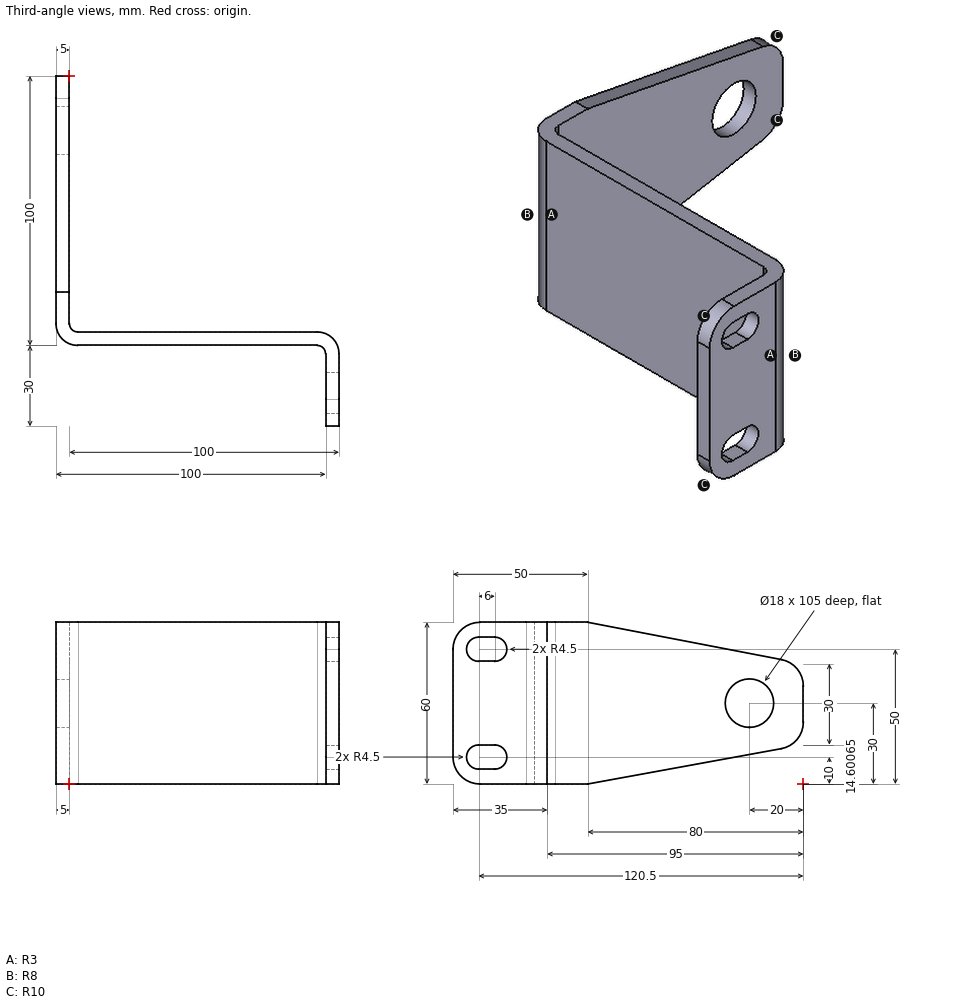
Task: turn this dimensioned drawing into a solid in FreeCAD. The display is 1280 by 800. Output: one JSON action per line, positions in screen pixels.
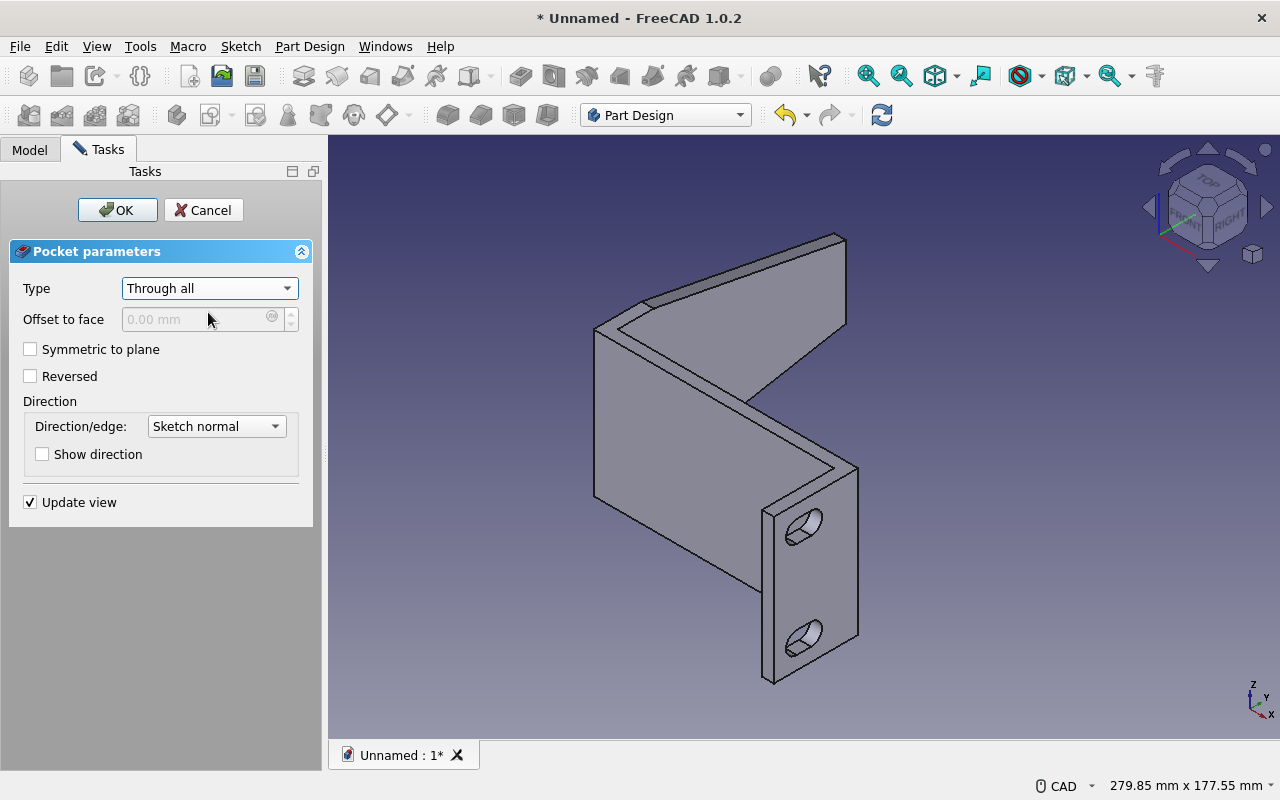
{"action": "left_click", "coordinate": [118, 210]}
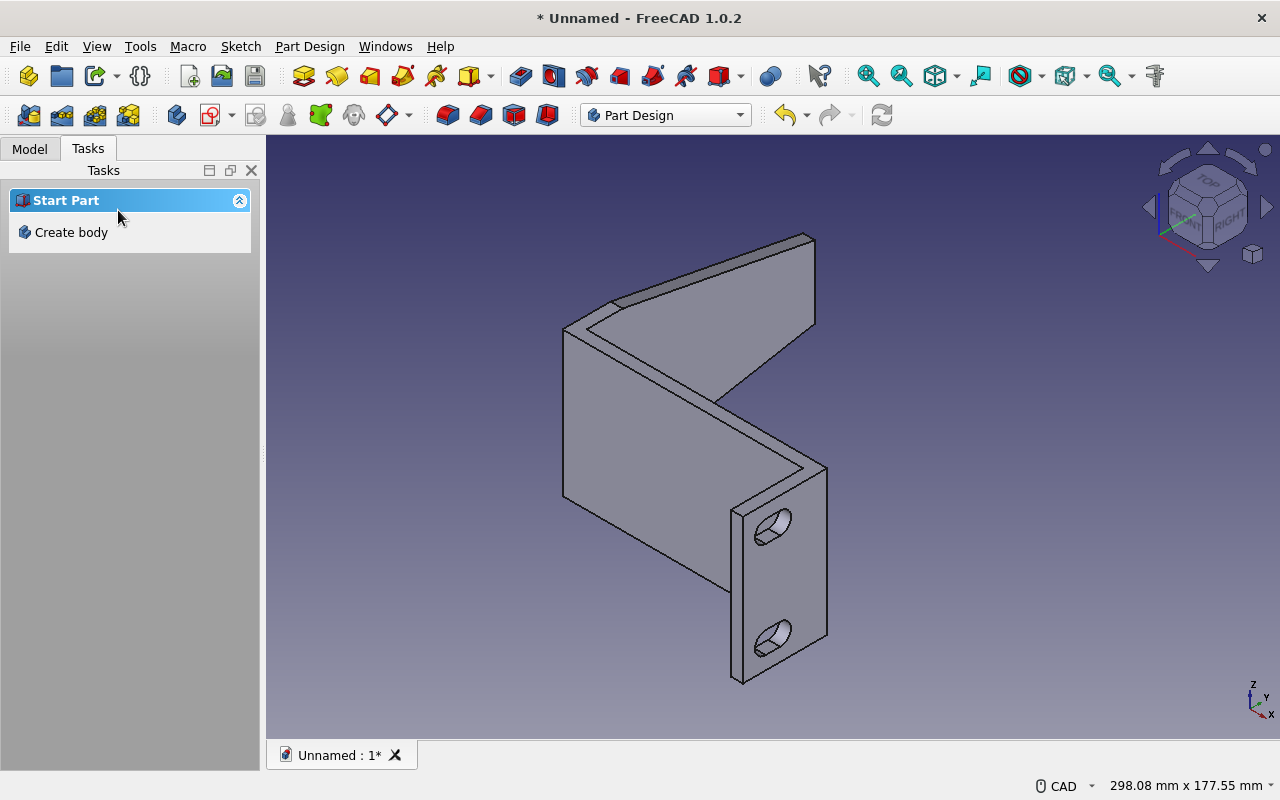
{"action": "key", "text": "6"}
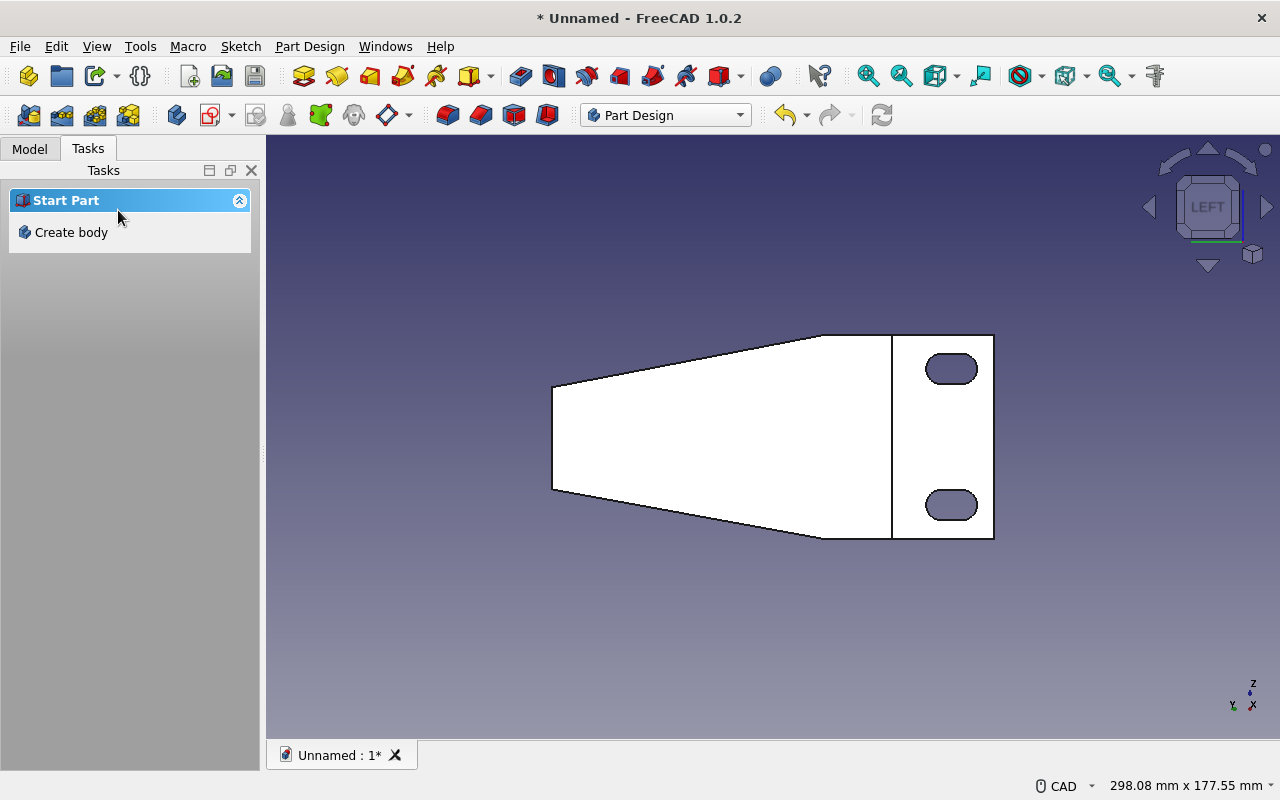
{"action": "left_click", "coordinate": [869, 76]}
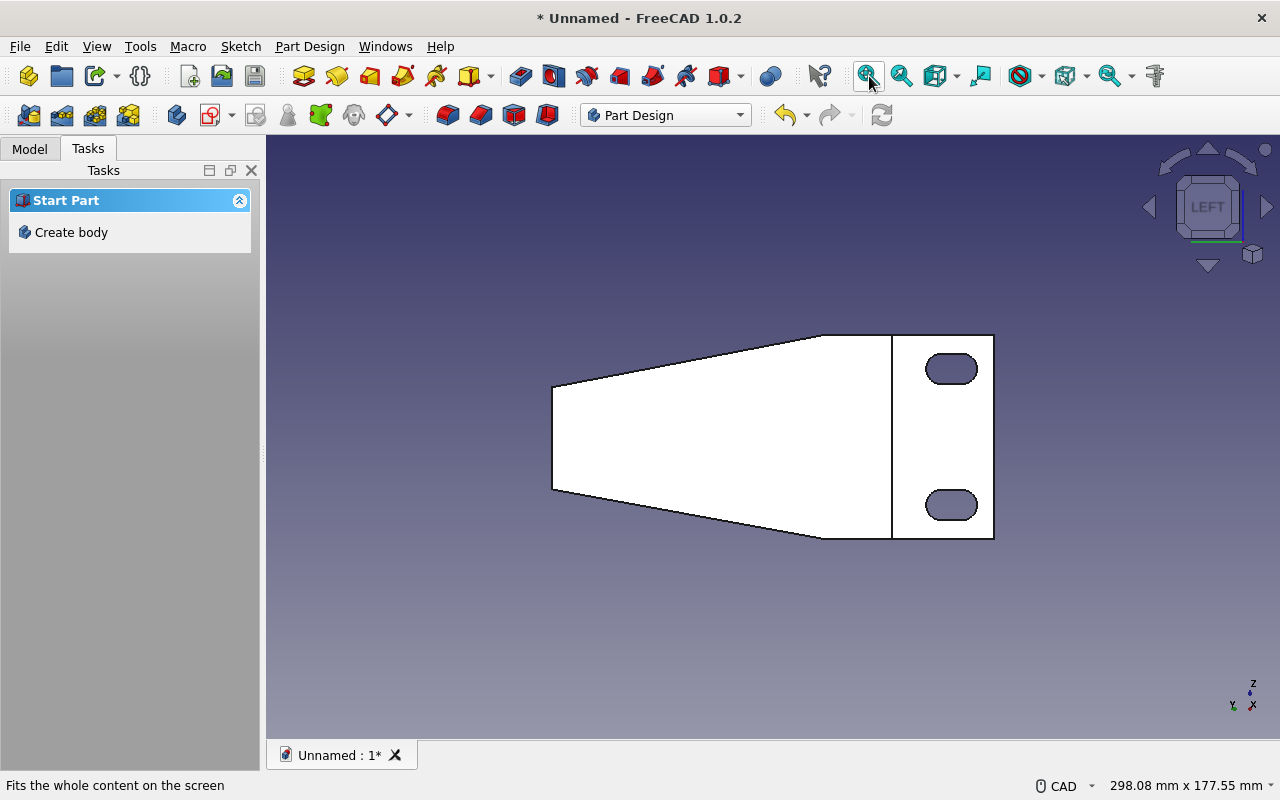
{"action": "left_click", "coordinate": [771, 436]}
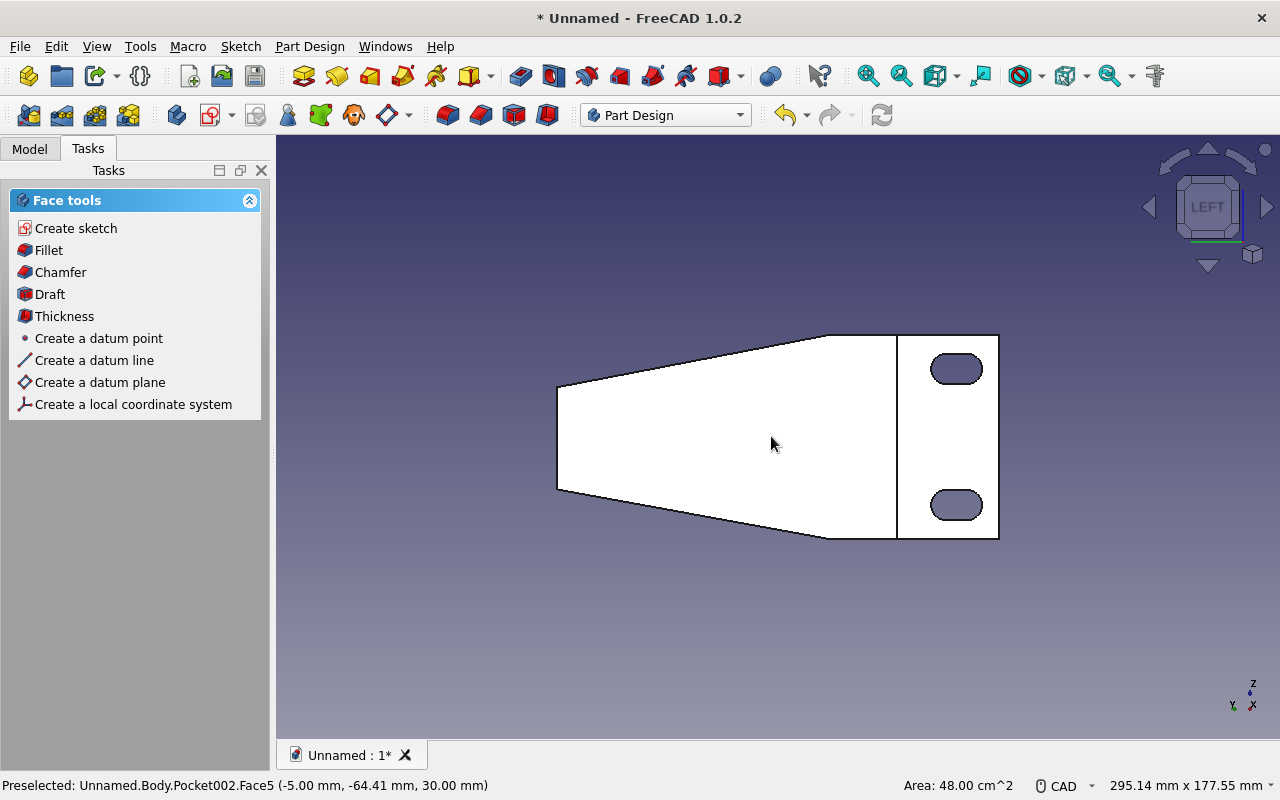
{"action": "left_click", "coordinate": [210, 116]}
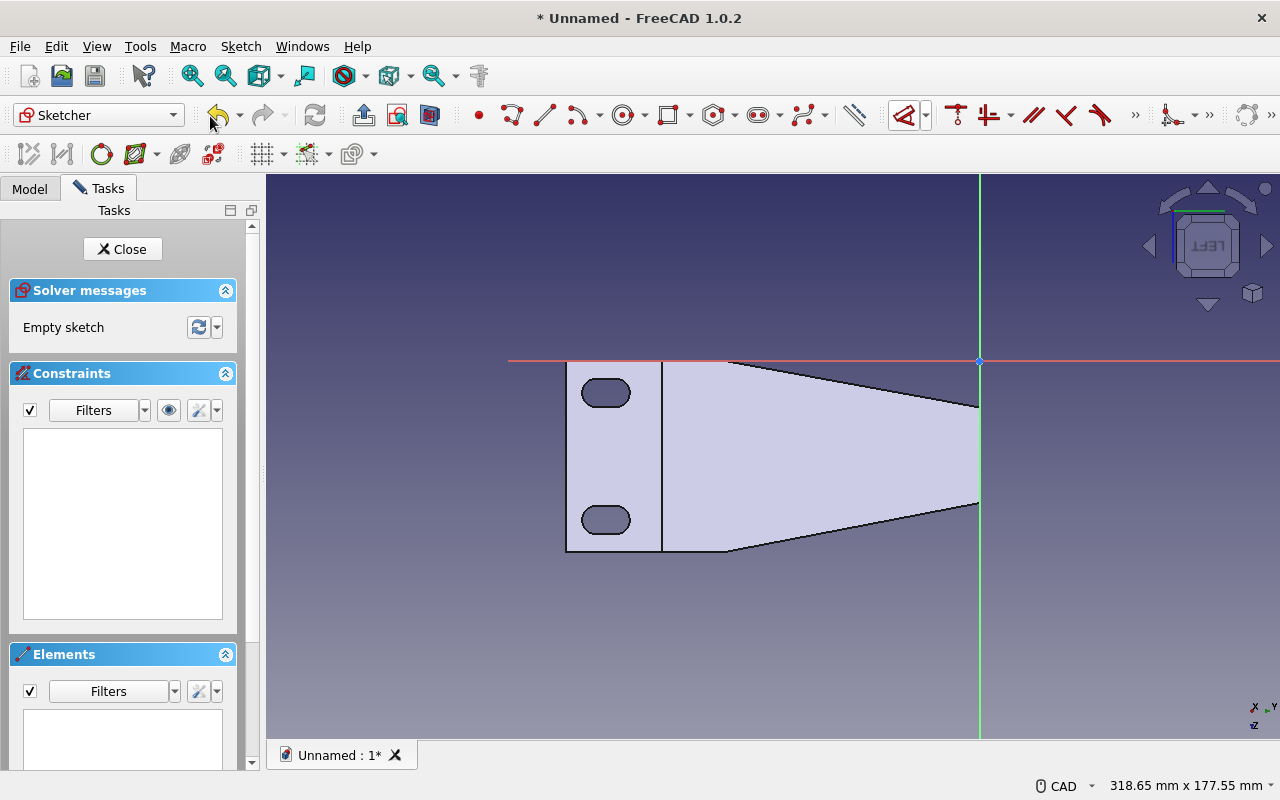
{"action": "scroll", "coordinate": [1067, 404], "scroll_direction": "up", "scroll_amount": 5}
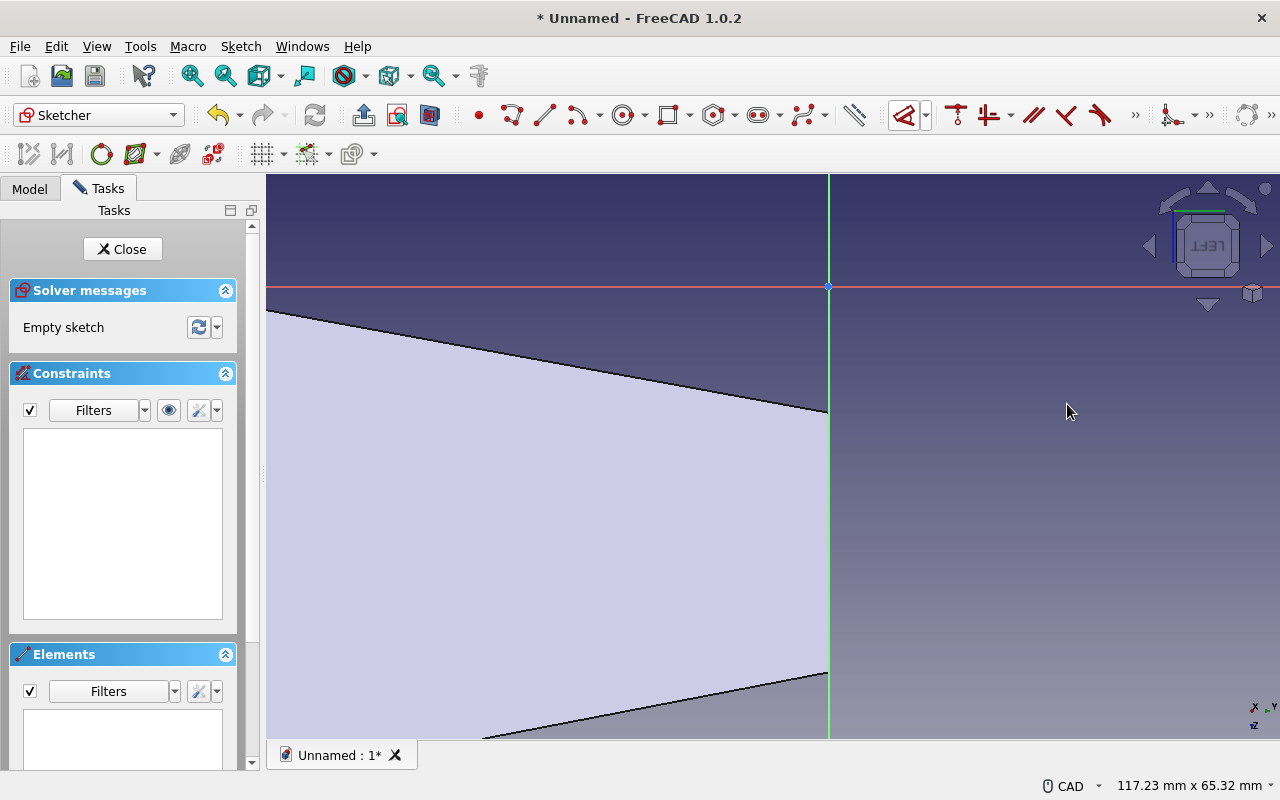
{"action": "left_click", "coordinate": [622, 116]}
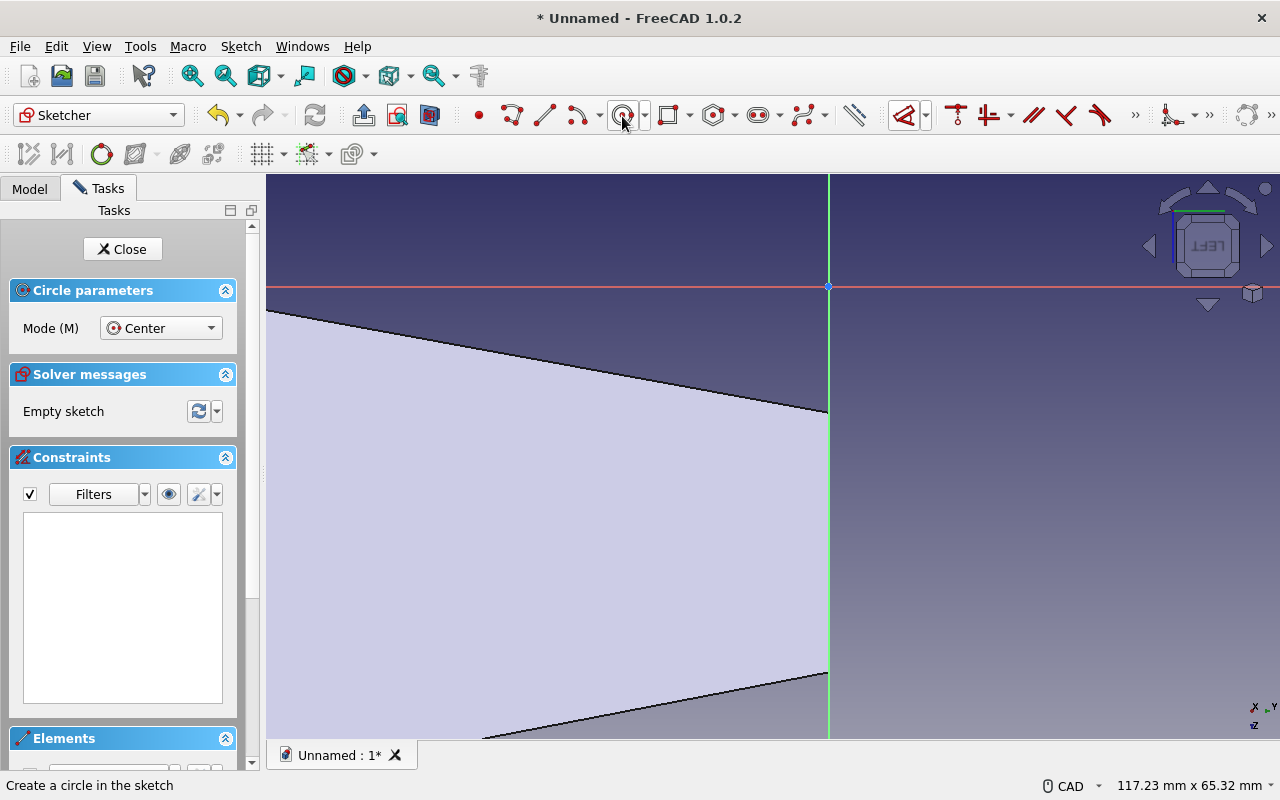
{"action": "left_click", "coordinate": [656, 546]}
{"action": "left_click", "coordinate": [711, 491]}
{"action": "key", "text": "Escape"}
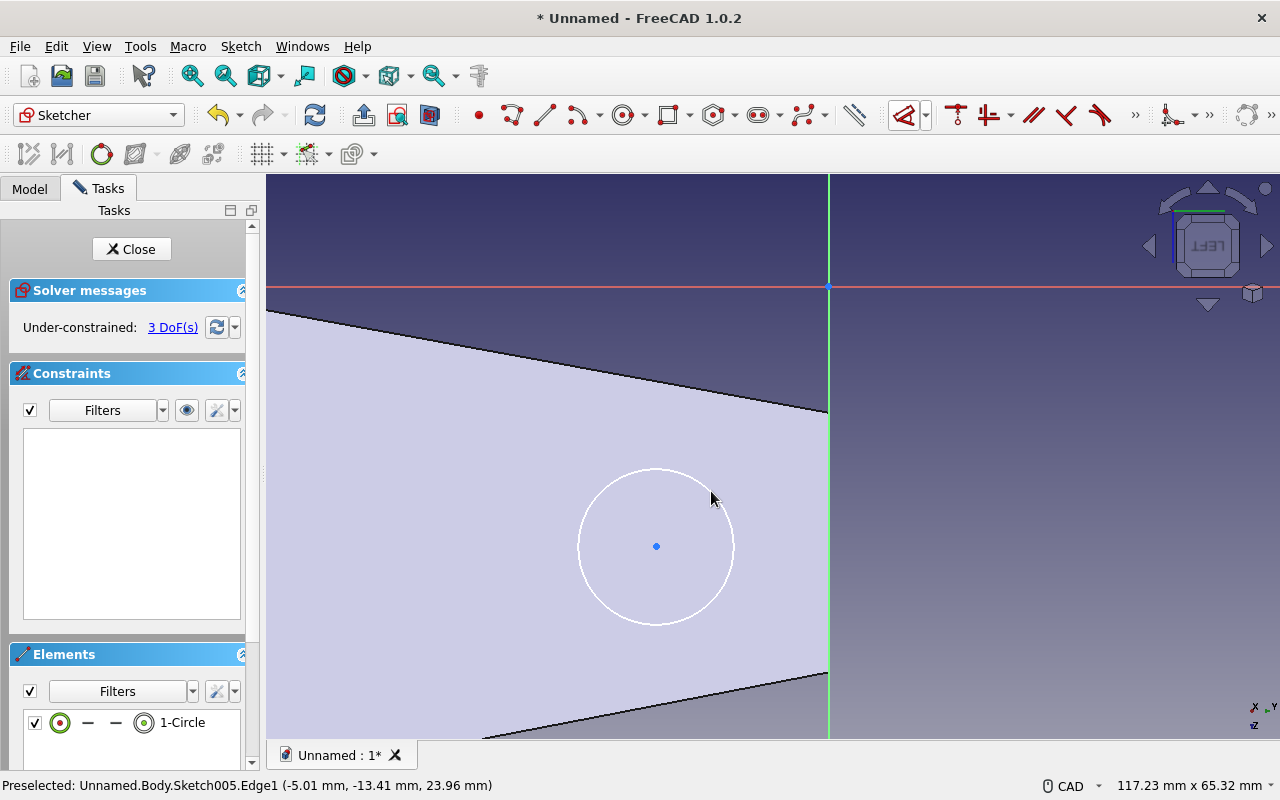
{"action": "left_click", "coordinate": [711, 492]}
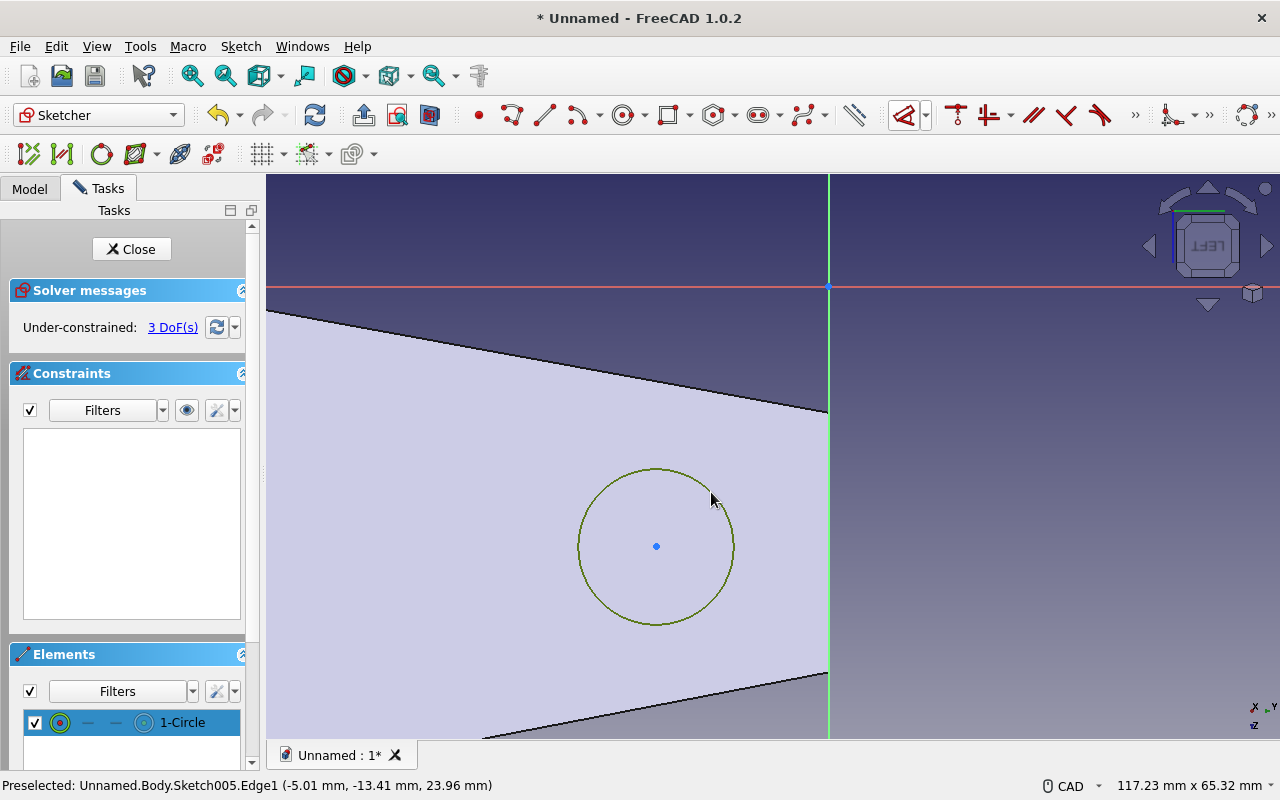
{"action": "left_click", "coordinate": [926, 116]}